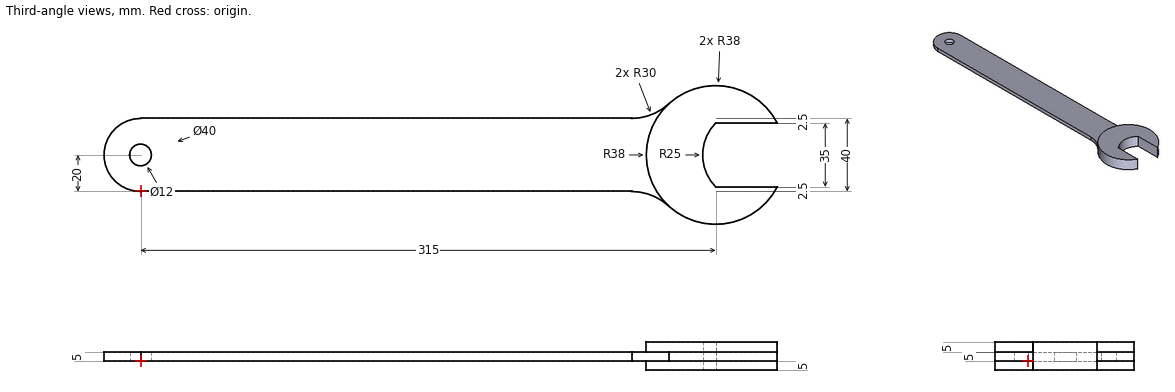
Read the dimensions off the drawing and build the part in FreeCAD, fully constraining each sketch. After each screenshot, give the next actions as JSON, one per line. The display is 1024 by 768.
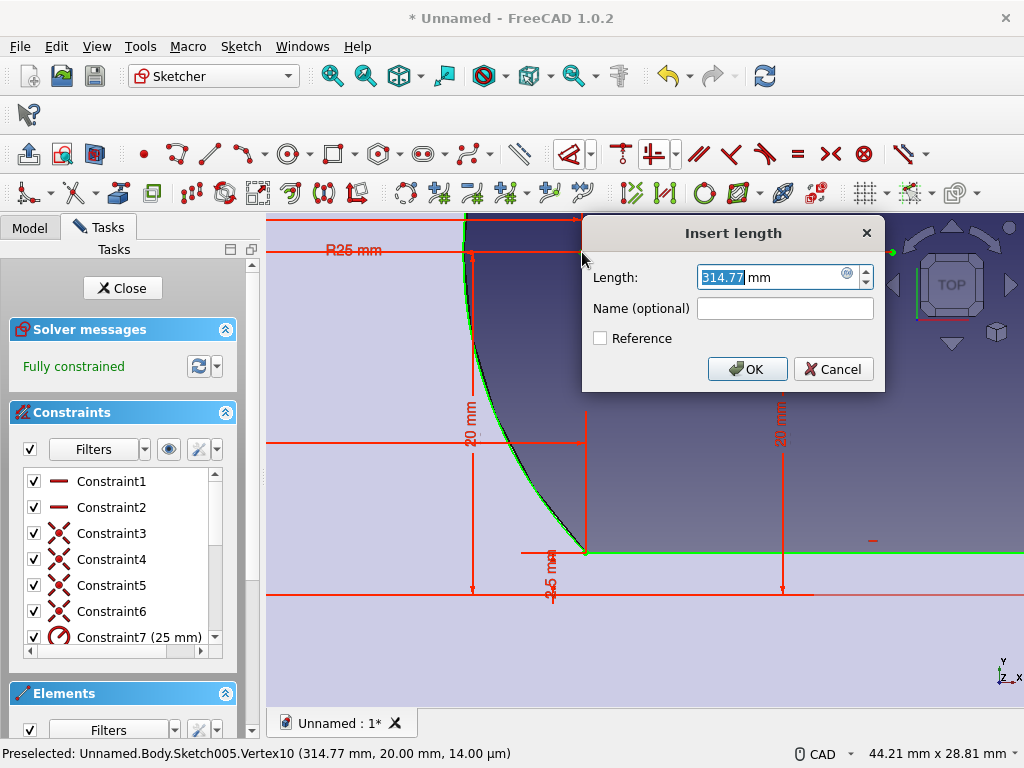
{"action": "type", "text": "315"}
{"action": "key", "text": "Return"}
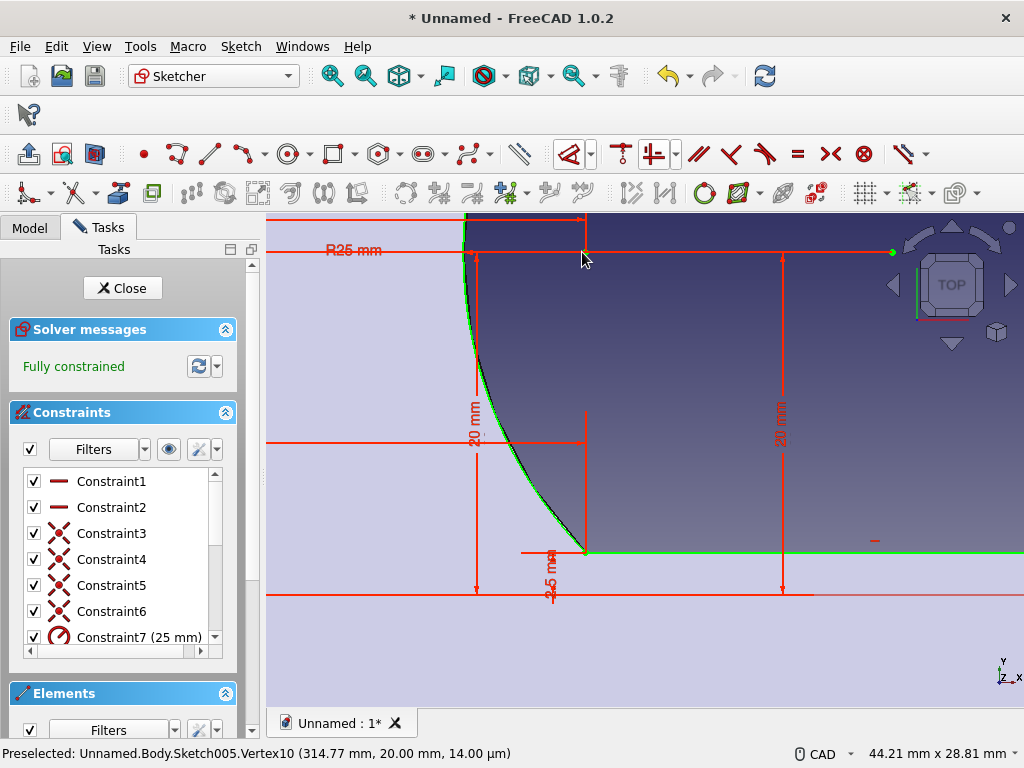
{"action": "left_click", "coordinate": [123, 288]}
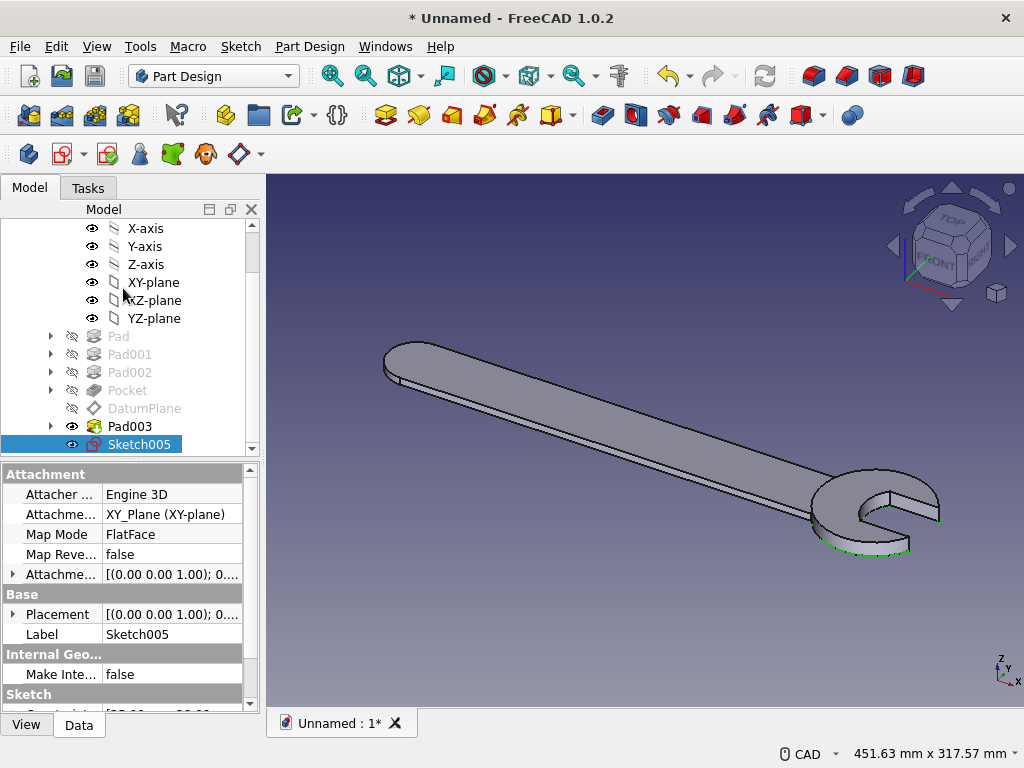
{"action": "left_click", "coordinate": [386, 116]}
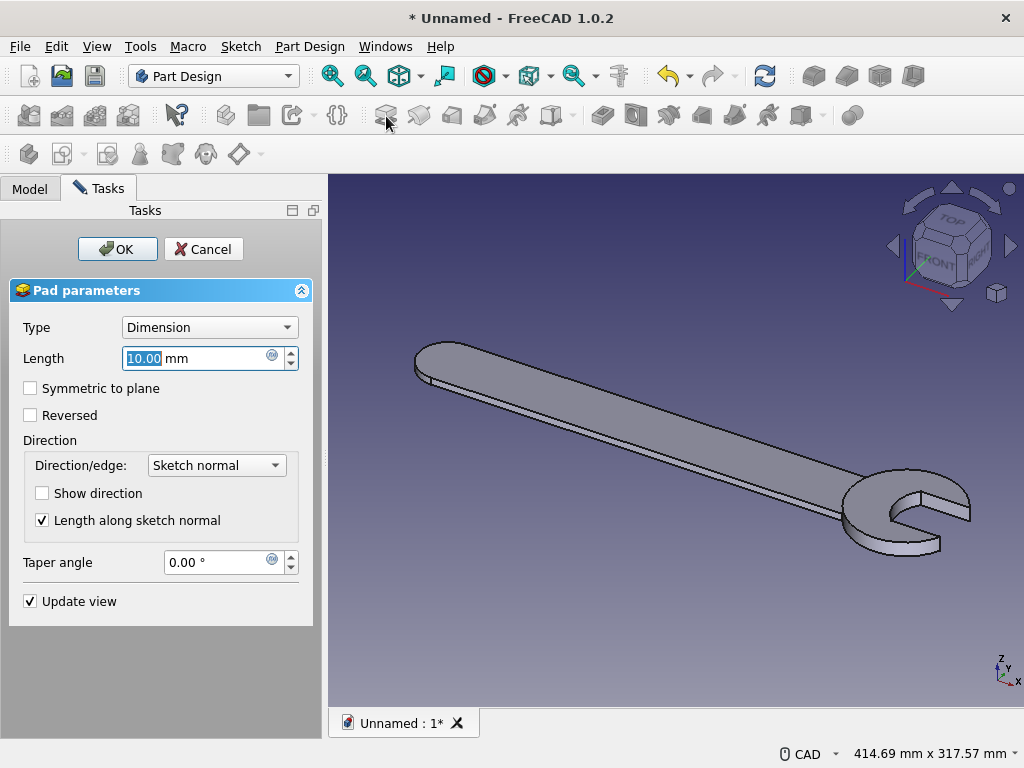
{"action": "type", "text": "5"}
{"action": "key", "text": "Tab"}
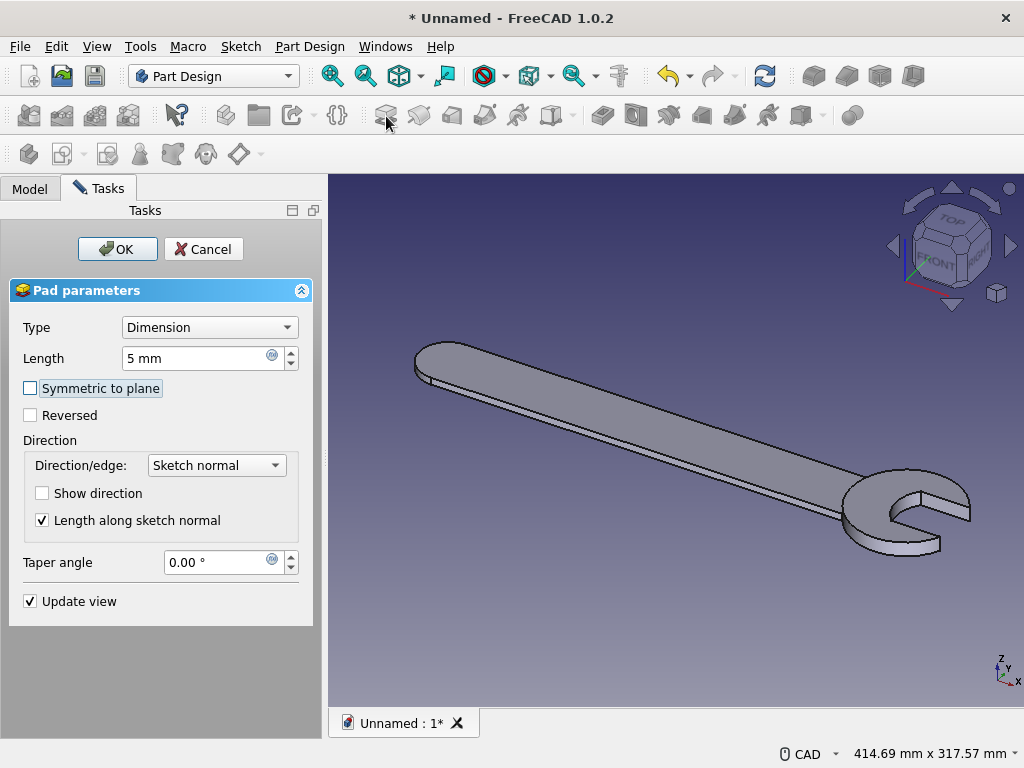
{"action": "left_click", "coordinate": [31, 415]}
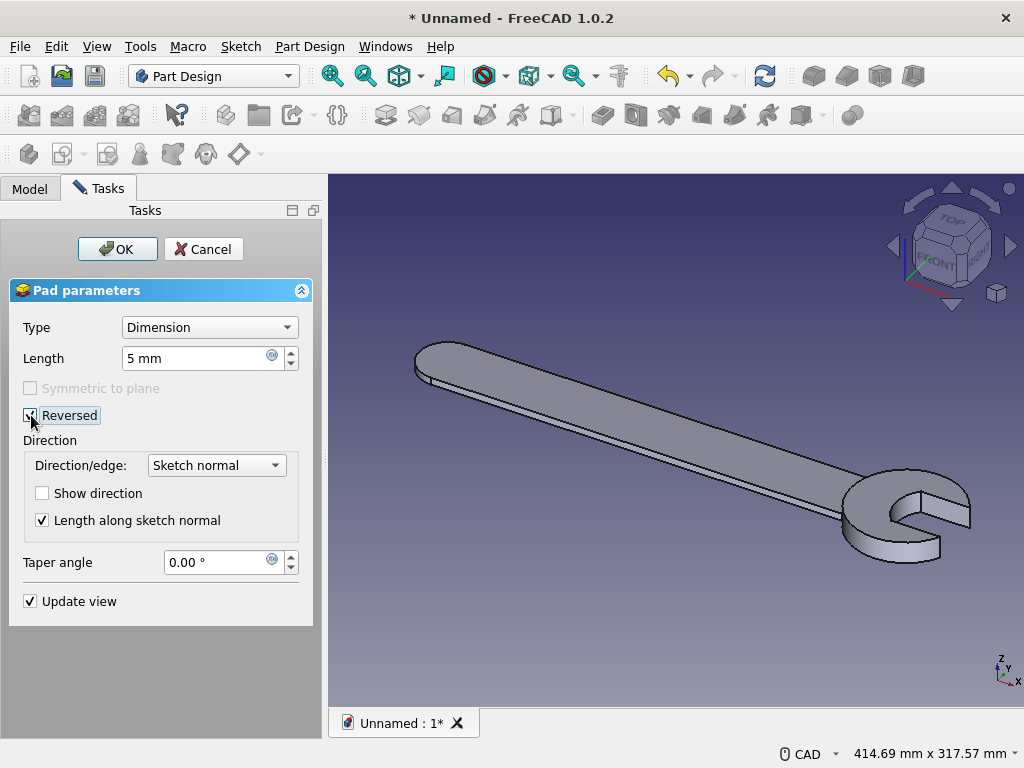
{"action": "left_click", "coordinate": [118, 249]}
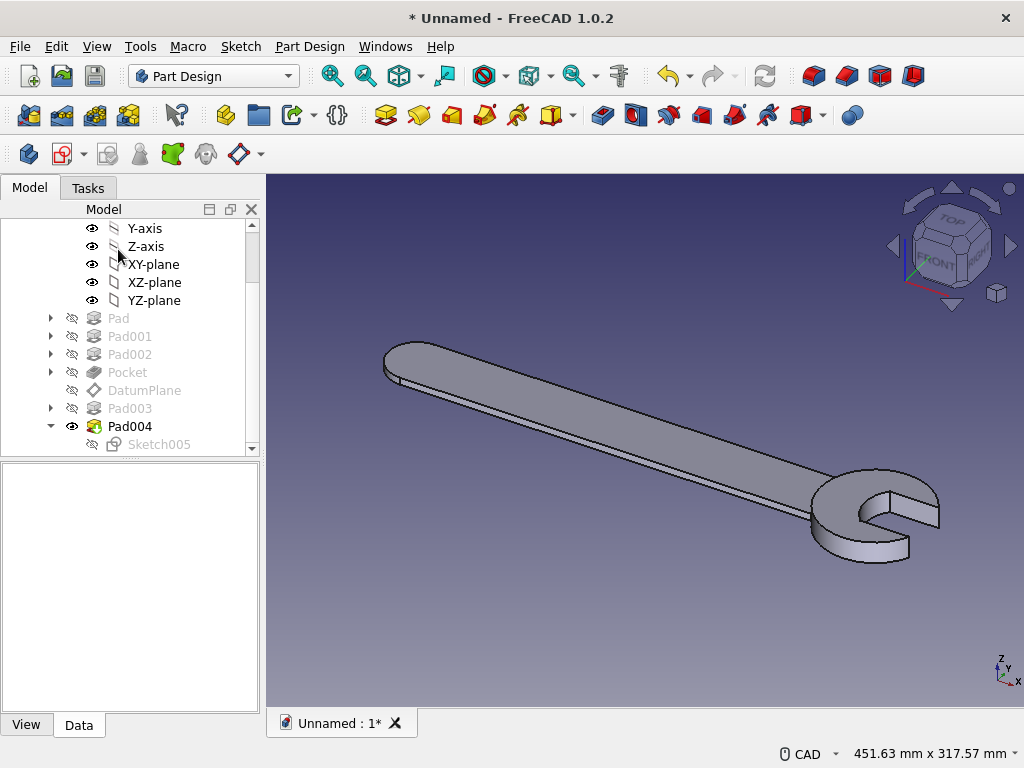
{"action": "left_click", "coordinate": [734, 465]}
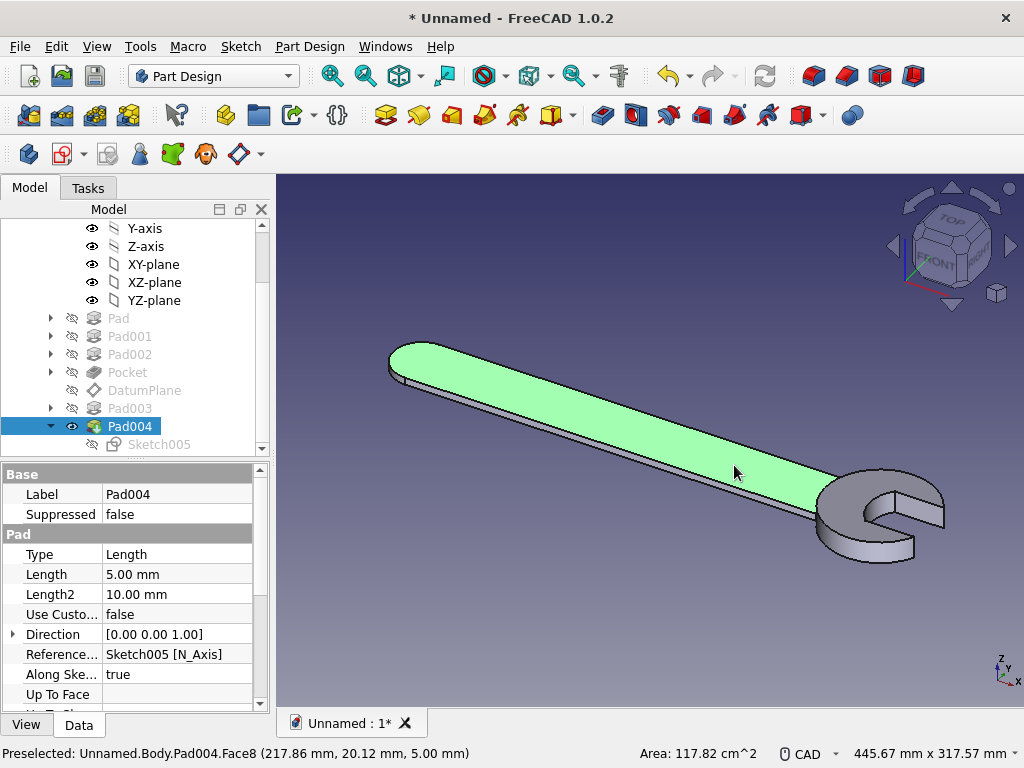
{"action": "left_click", "coordinate": [62, 154]}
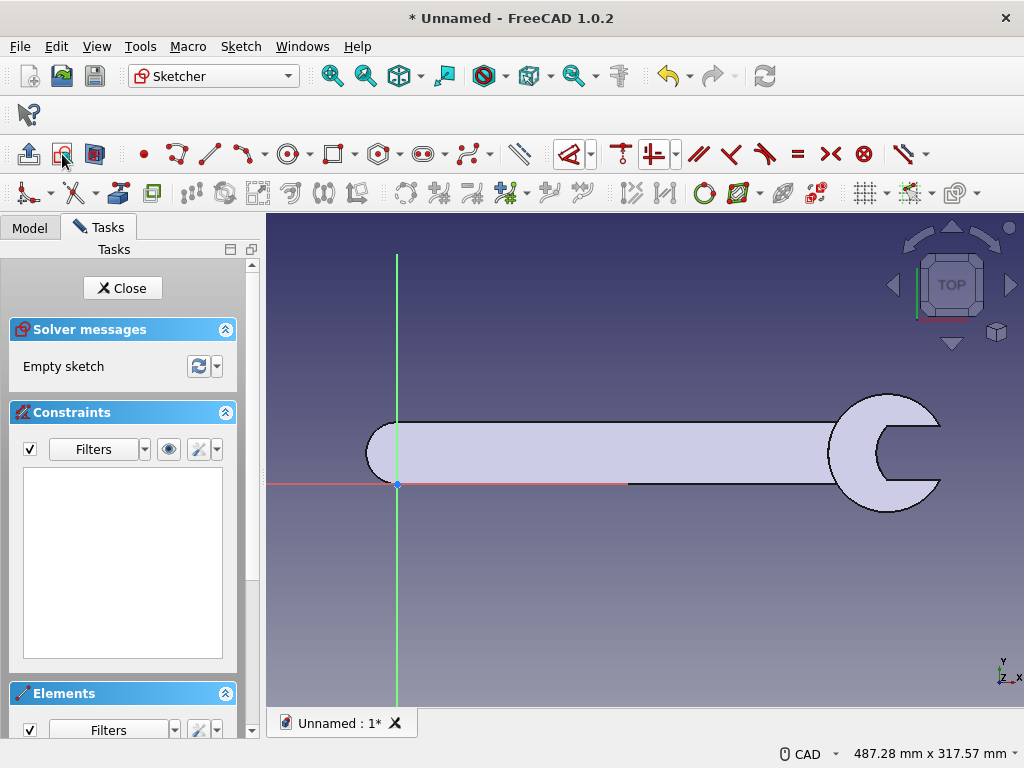
{"action": "left_click", "coordinate": [95, 154]}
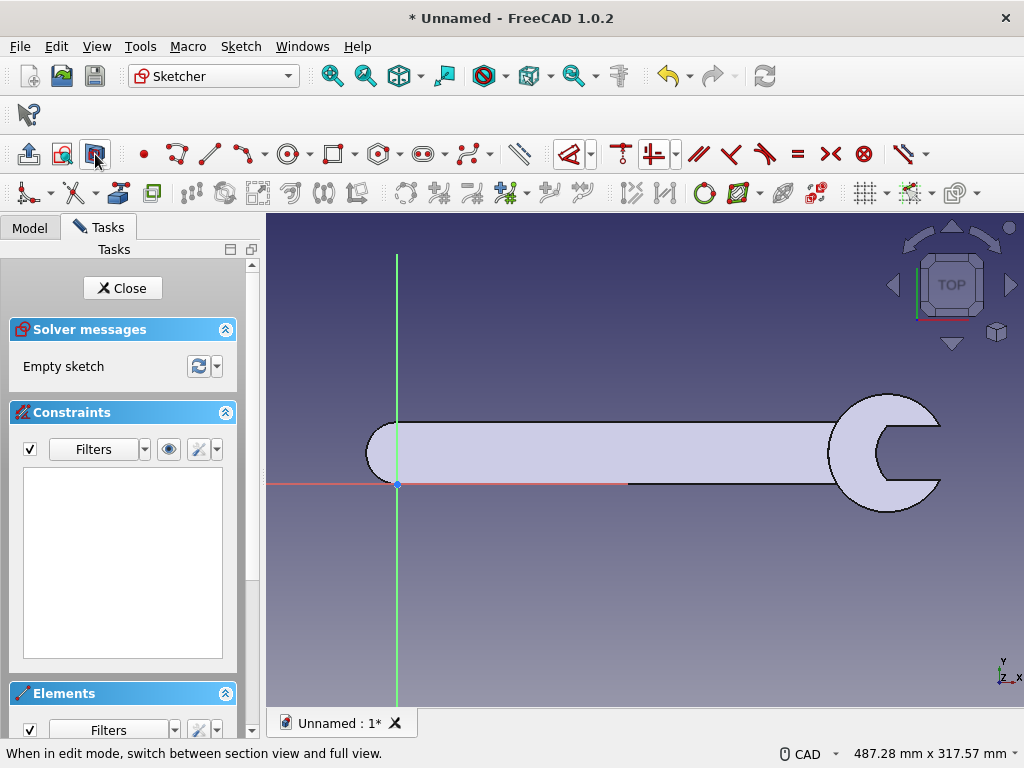
{"action": "scroll", "coordinate": [859, 450], "scroll_direction": "up", "scroll_amount": 6}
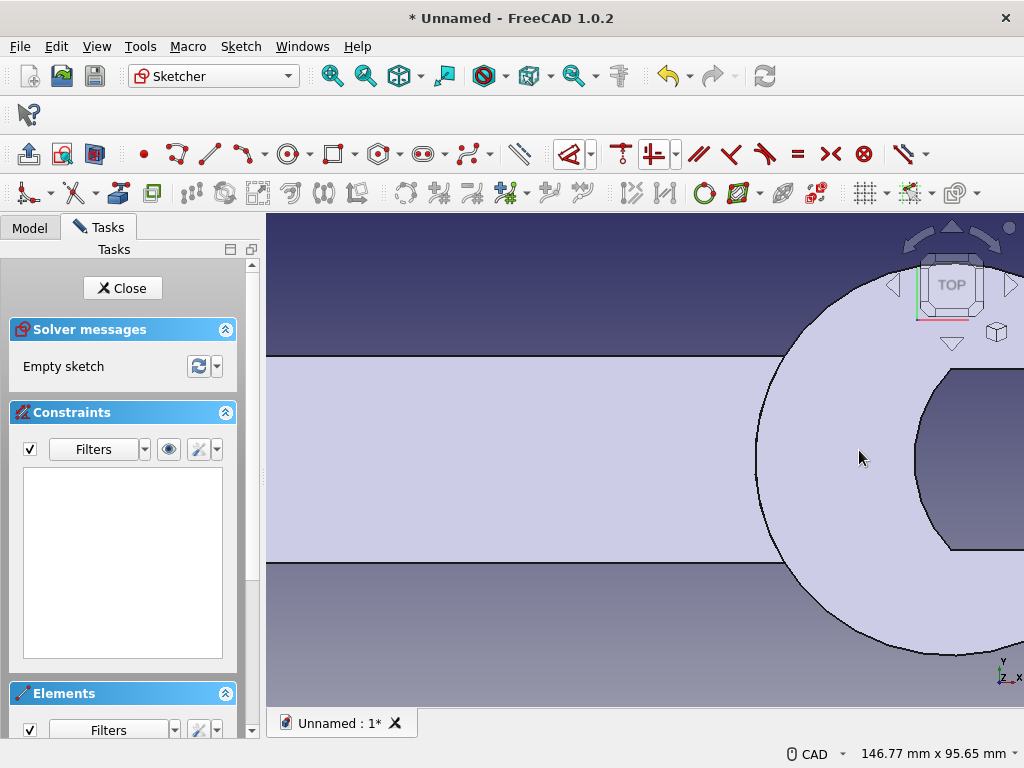
{"action": "left_click", "coordinate": [210, 154]}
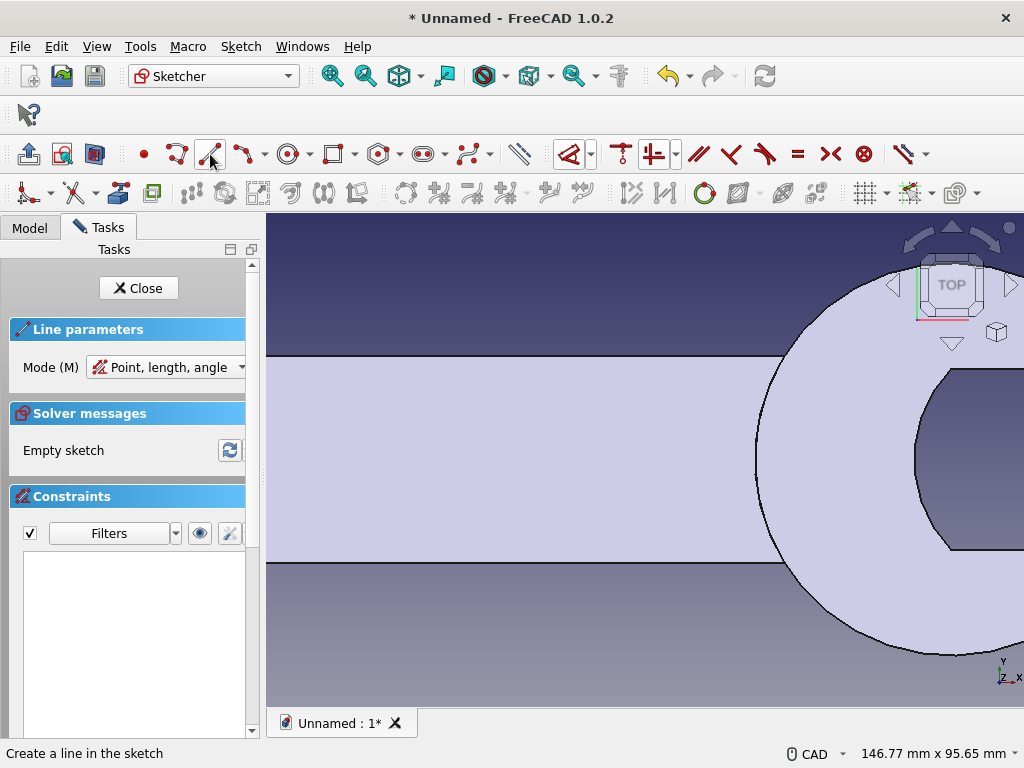
{"action": "left_click", "coordinate": [784, 356]}
{"action": "left_click", "coordinate": [713, 356]}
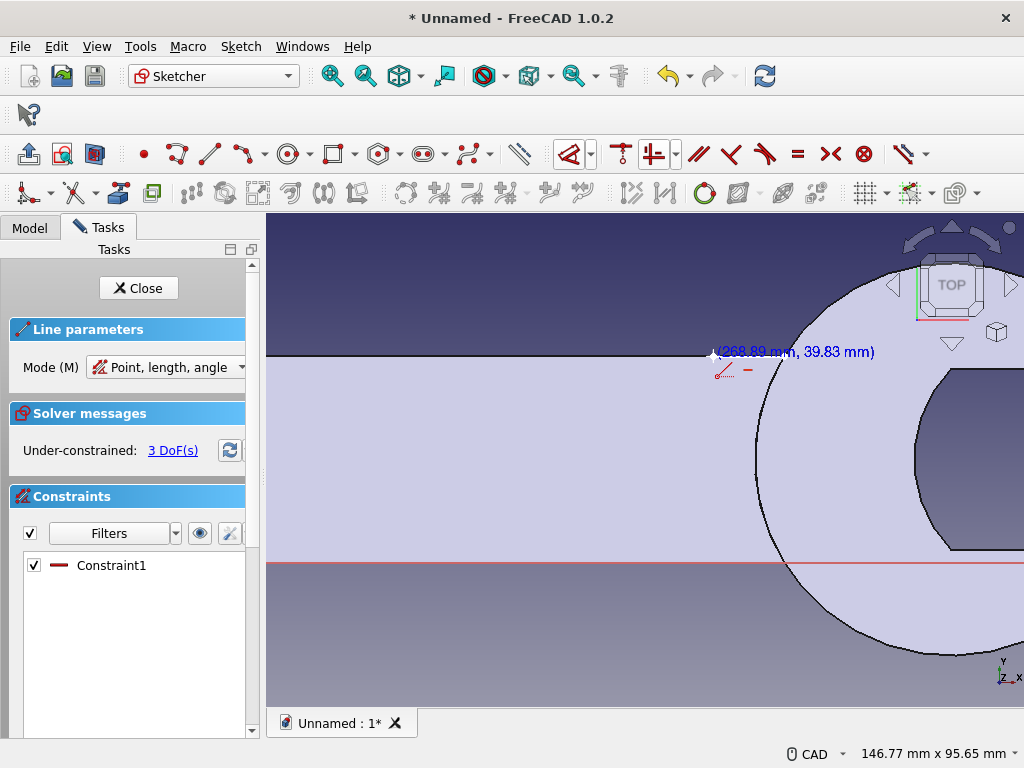
{"action": "left_click", "coordinate": [242, 154]}